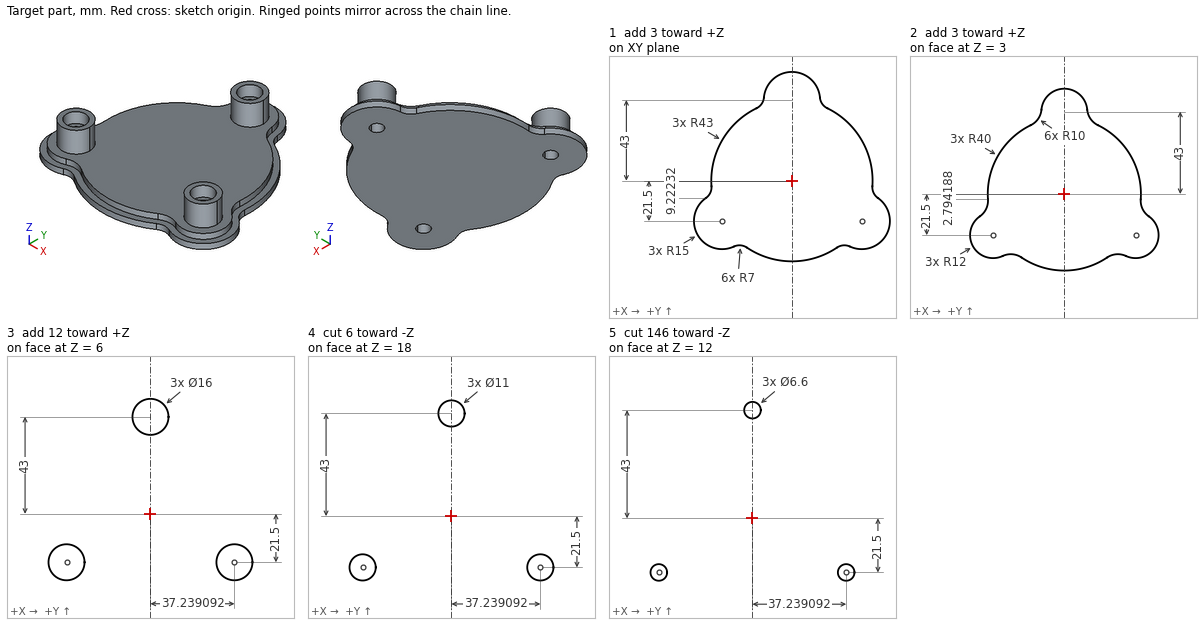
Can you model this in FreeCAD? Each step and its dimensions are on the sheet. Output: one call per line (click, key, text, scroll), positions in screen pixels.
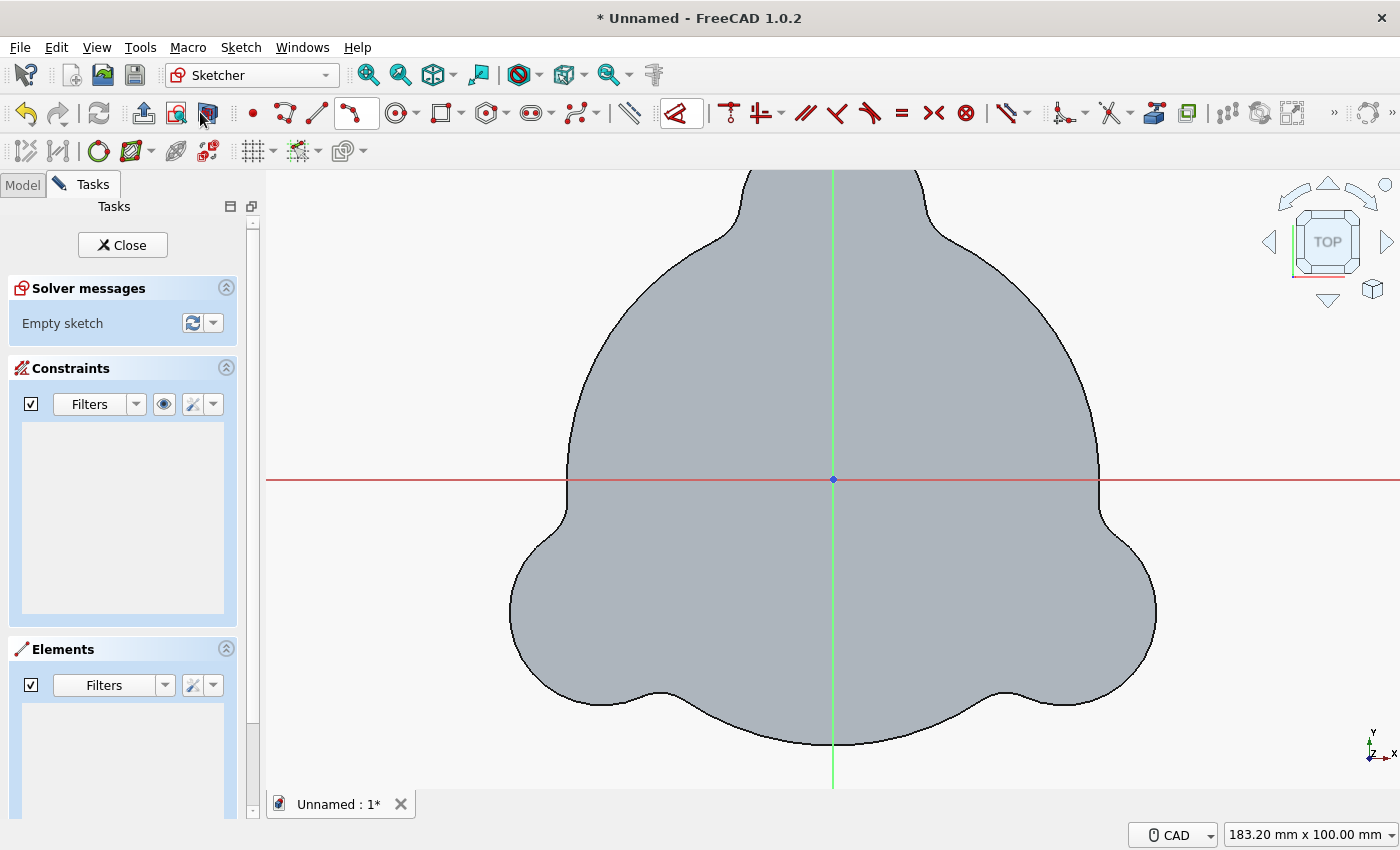
scroll(625, 574, down, 2)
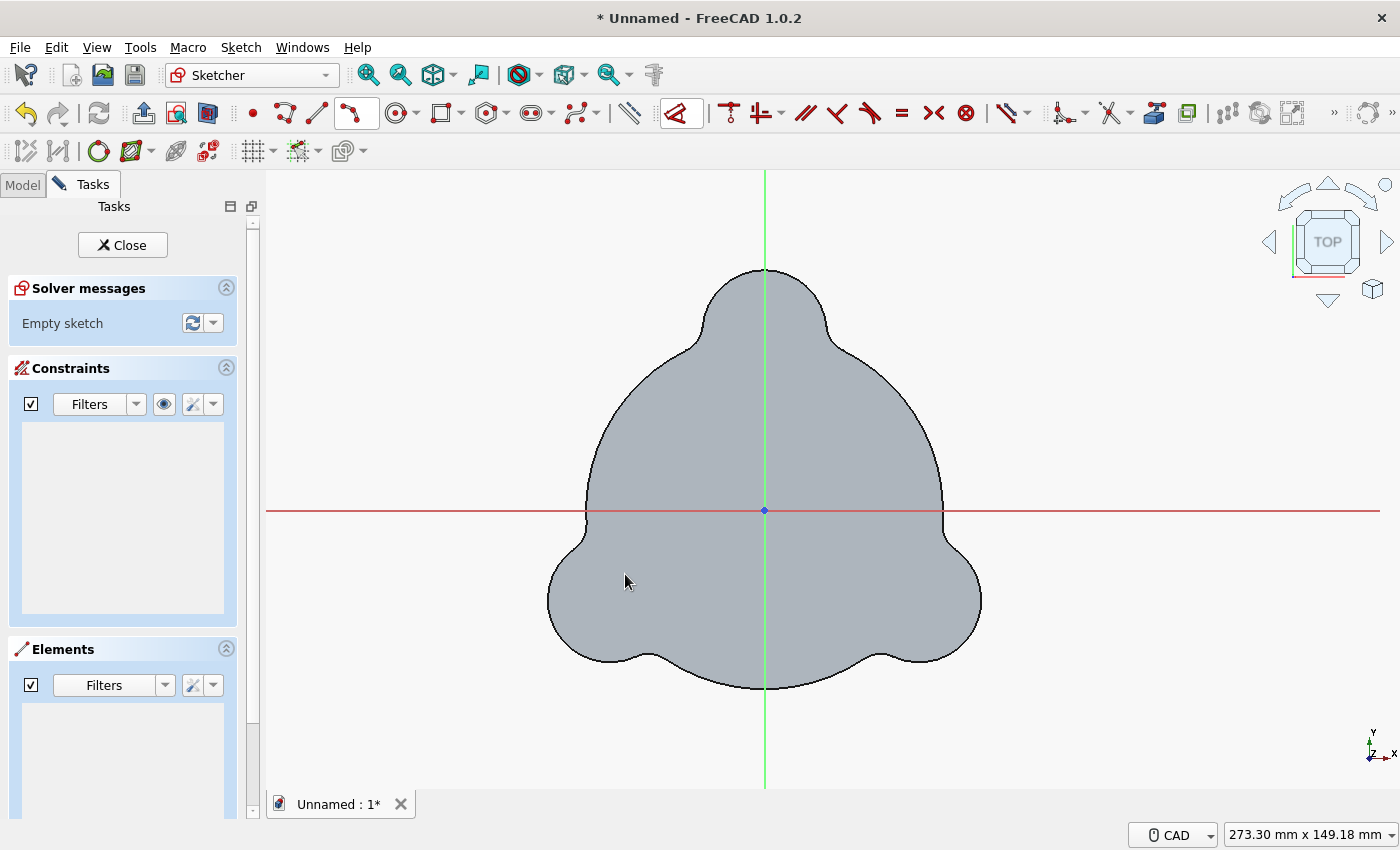
click(350, 114)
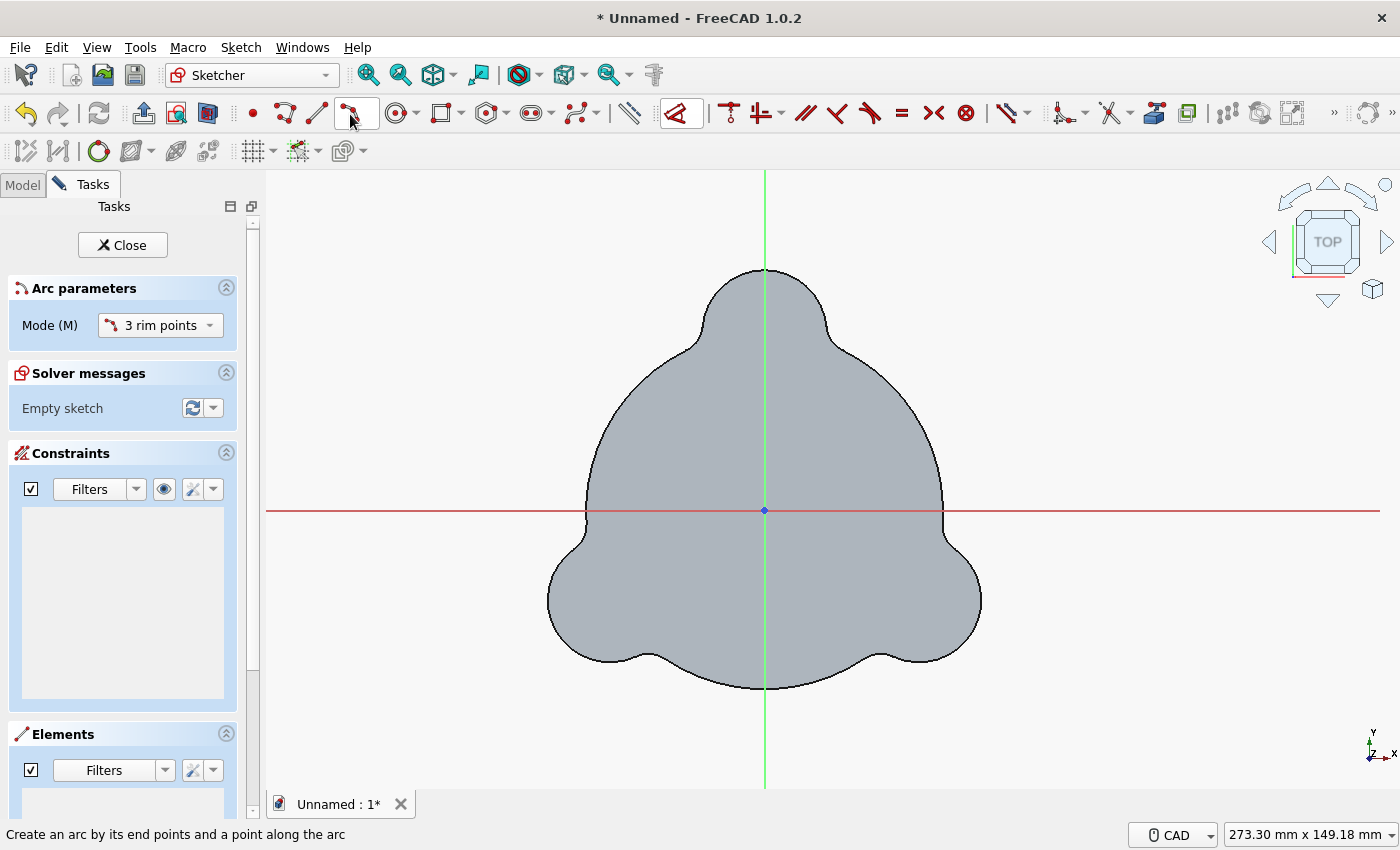
click(692, 362)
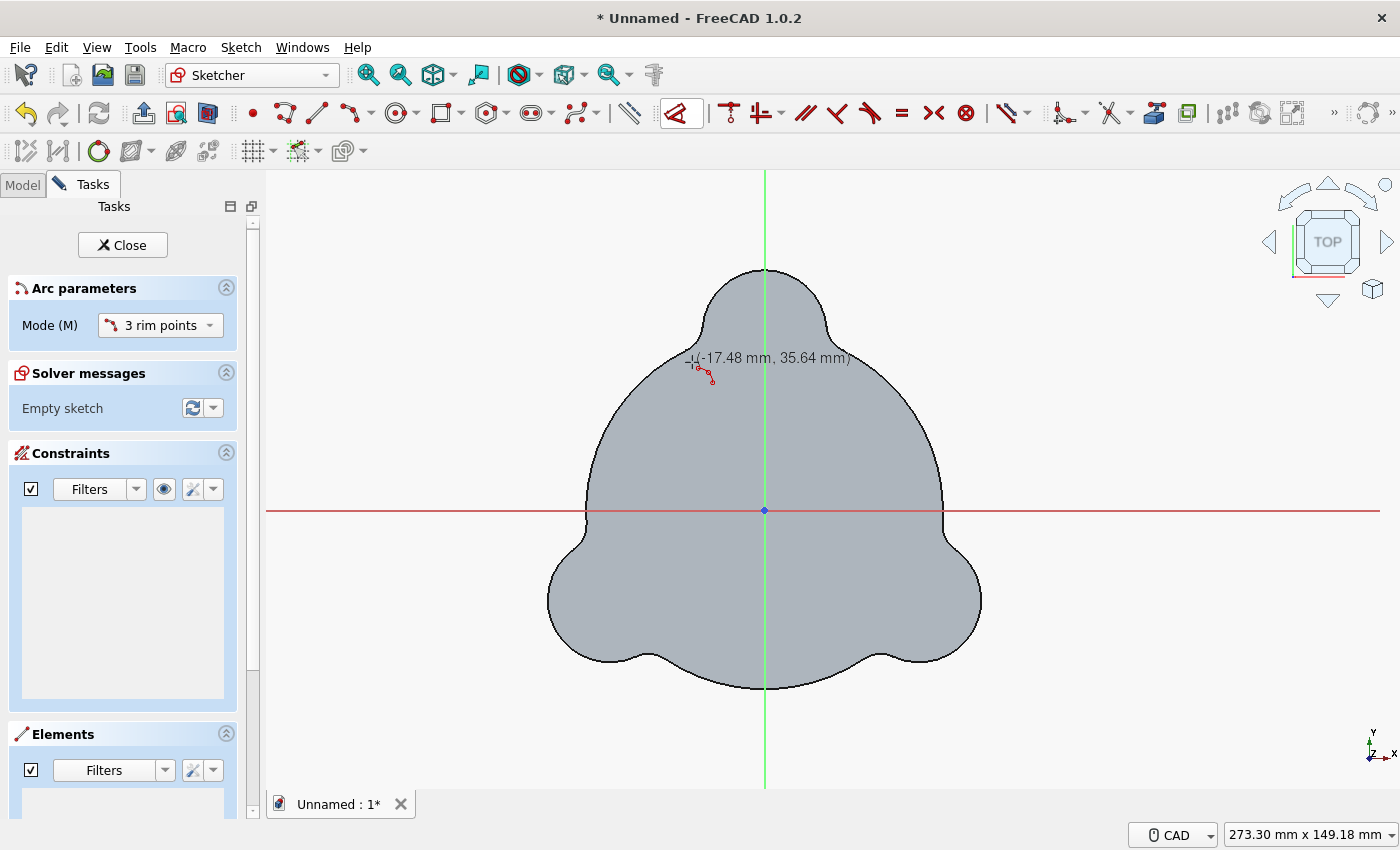
scroll(599, 522, up, 2)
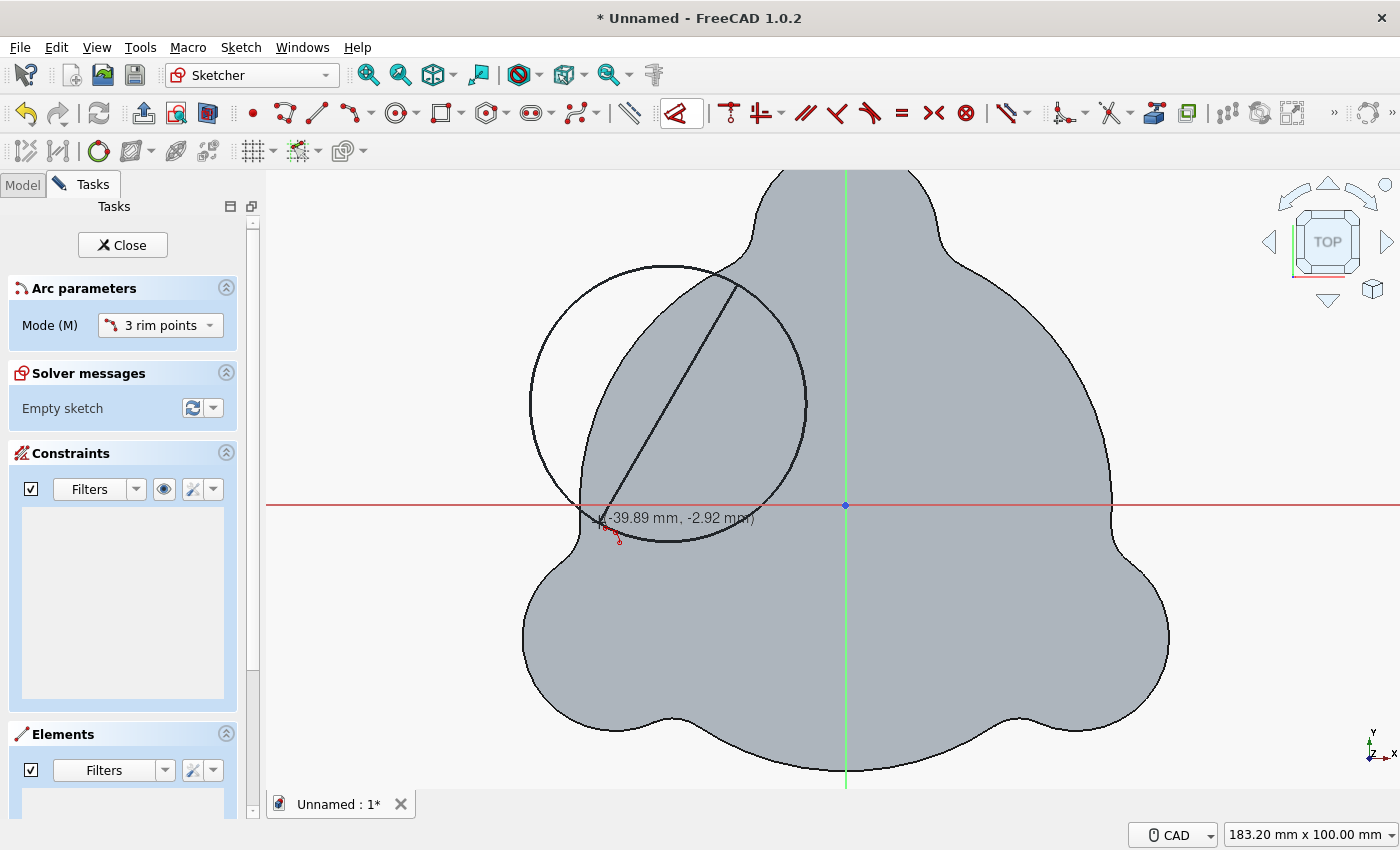
click(599, 522)
click(631, 381)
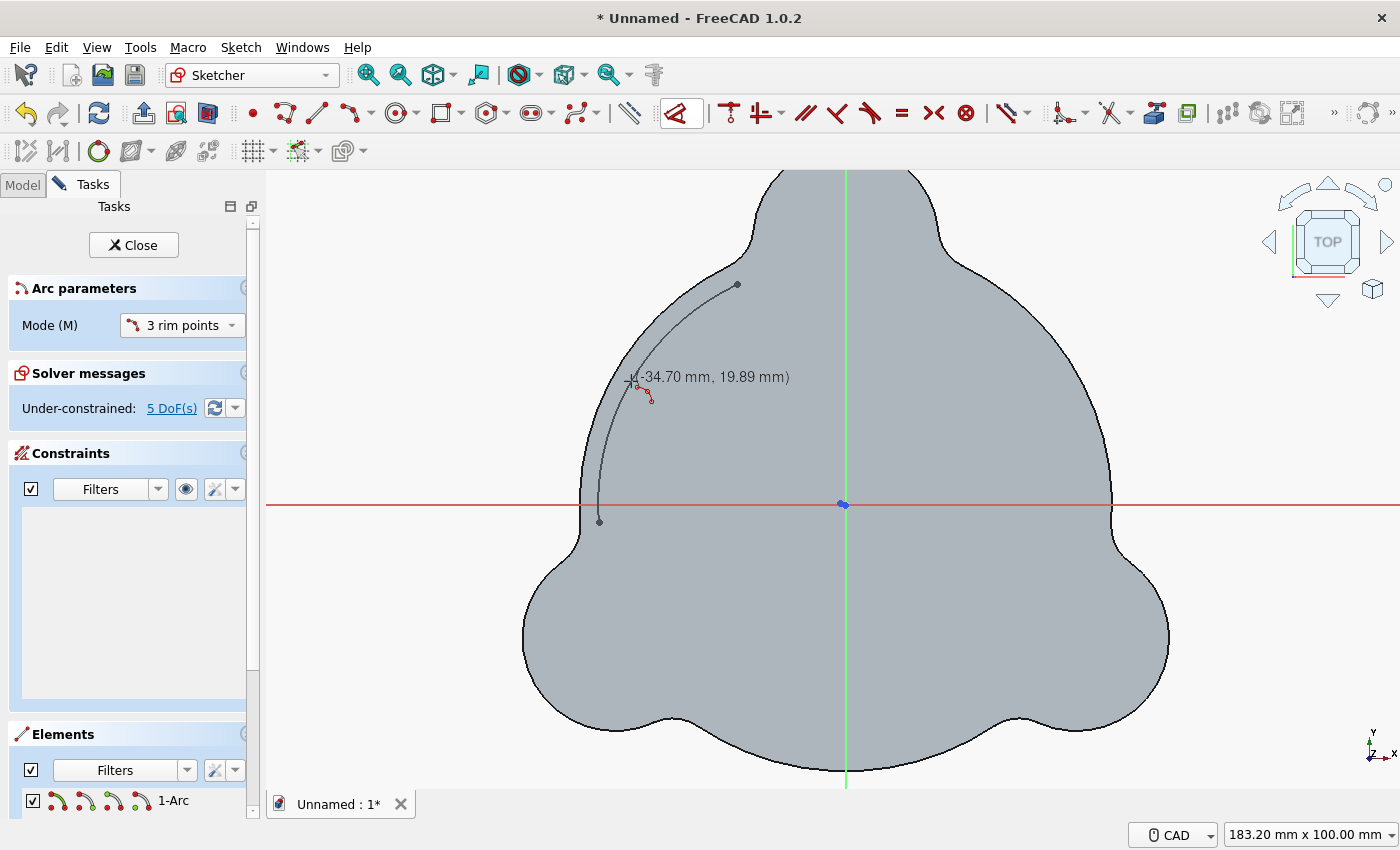
click(599, 523)
click(573, 577)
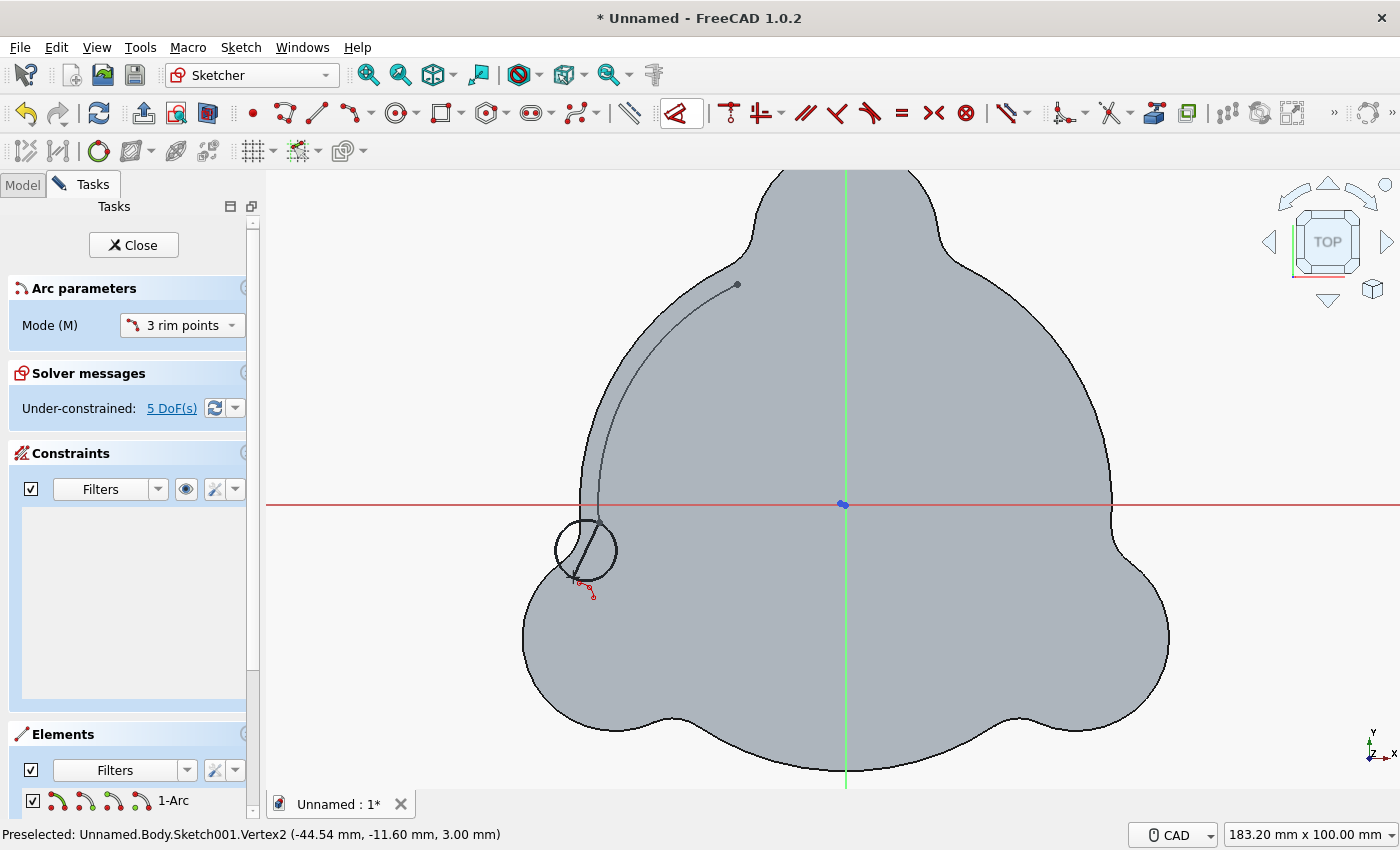
scroll(593, 553, up, 4)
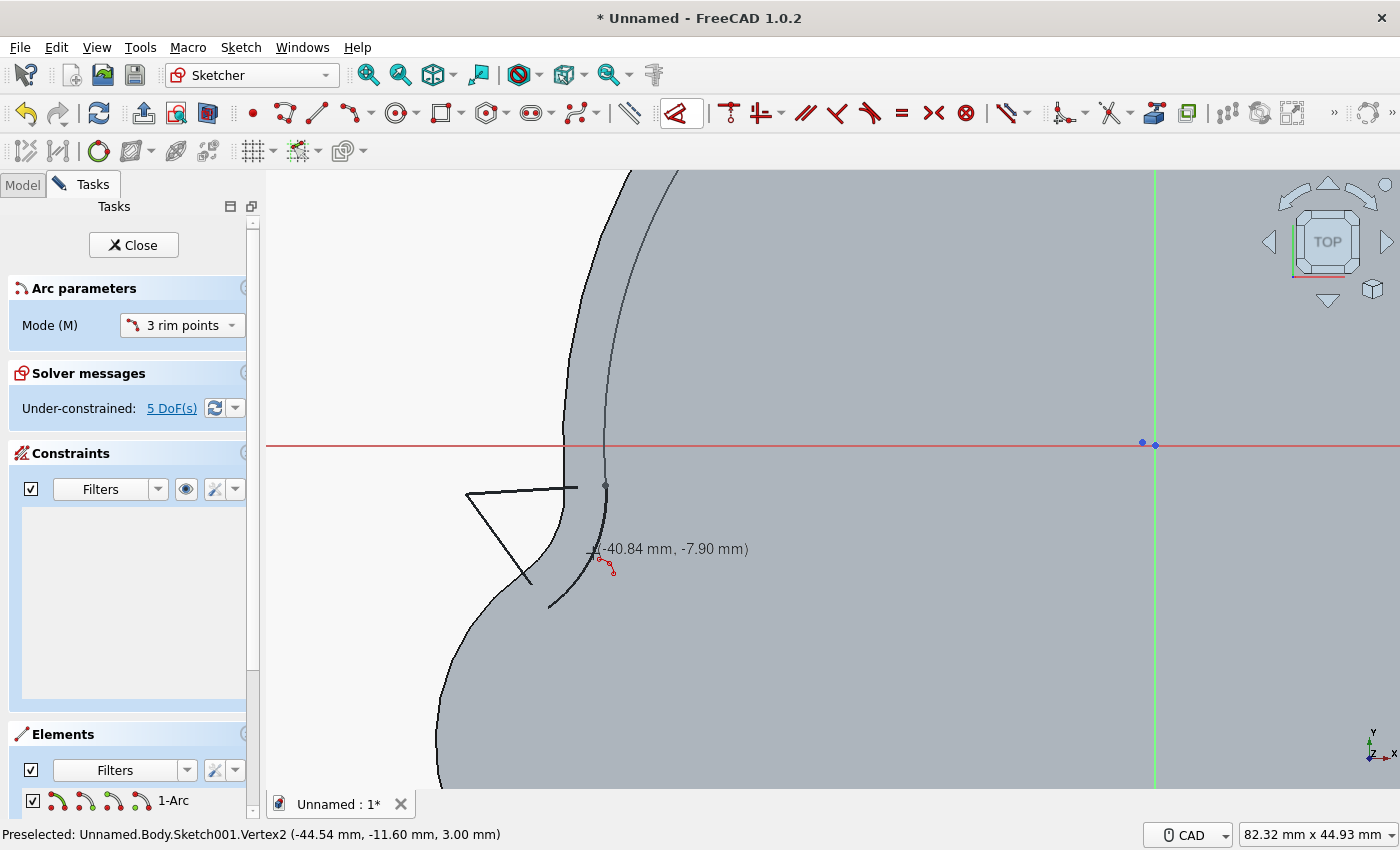
click(593, 553)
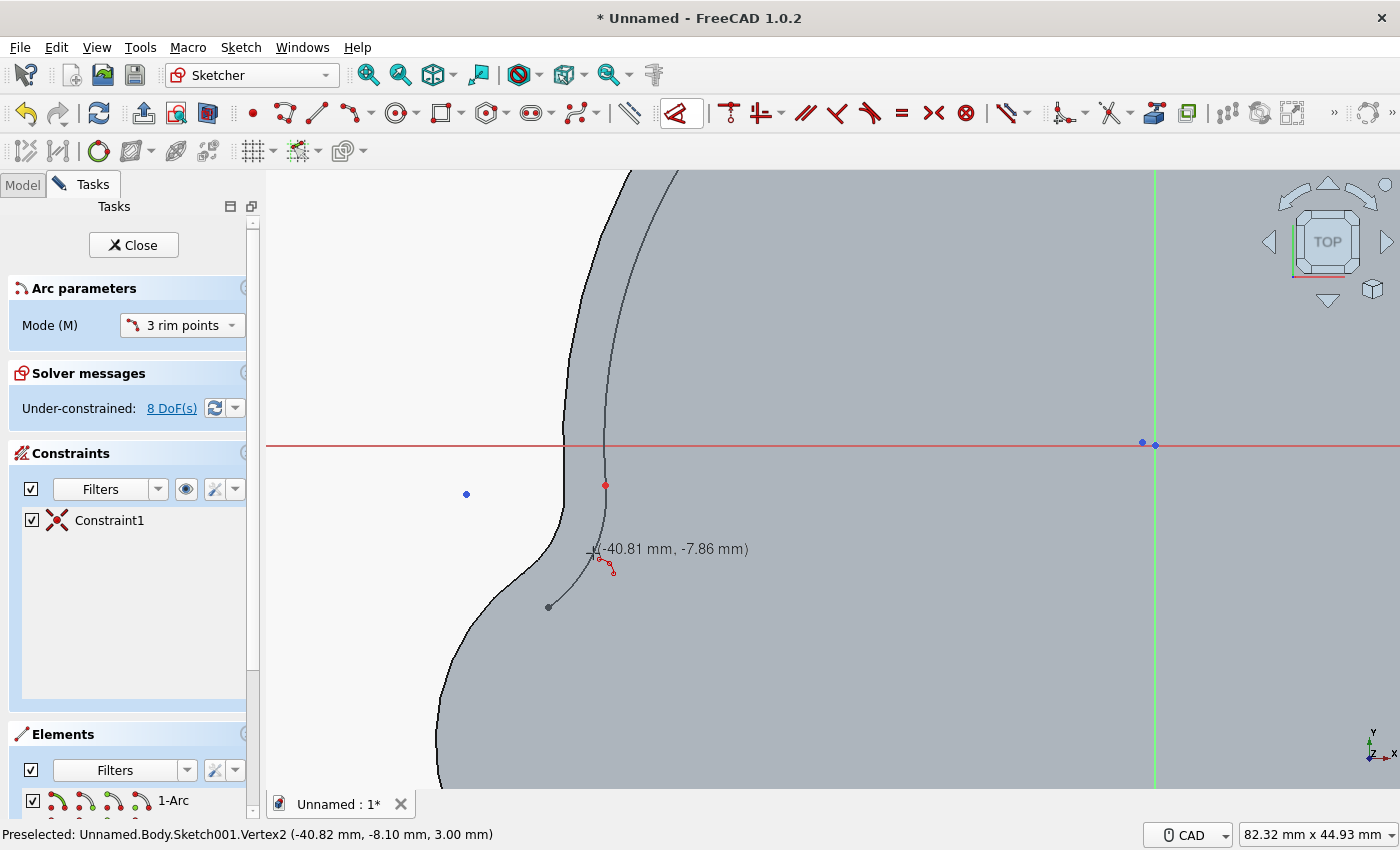
click(548, 608)